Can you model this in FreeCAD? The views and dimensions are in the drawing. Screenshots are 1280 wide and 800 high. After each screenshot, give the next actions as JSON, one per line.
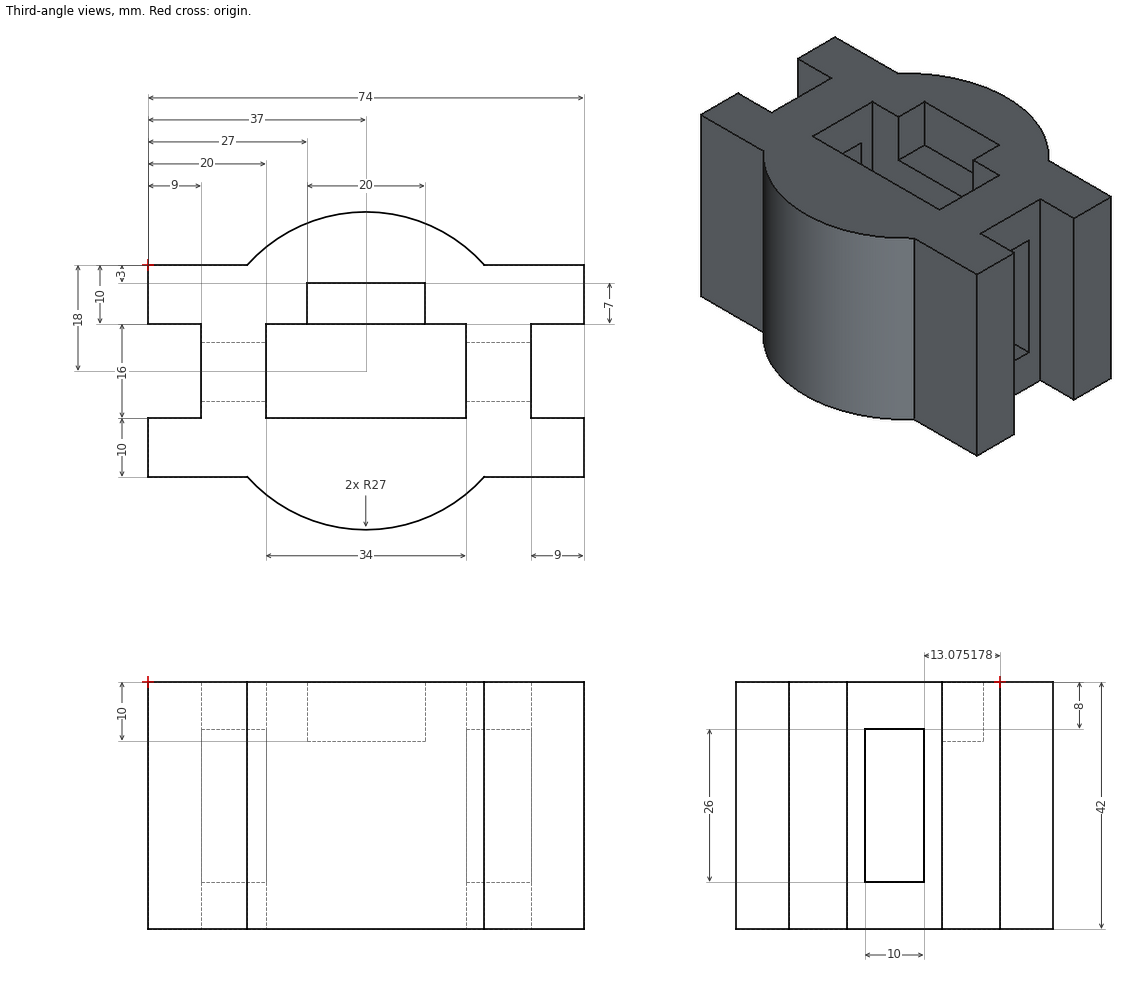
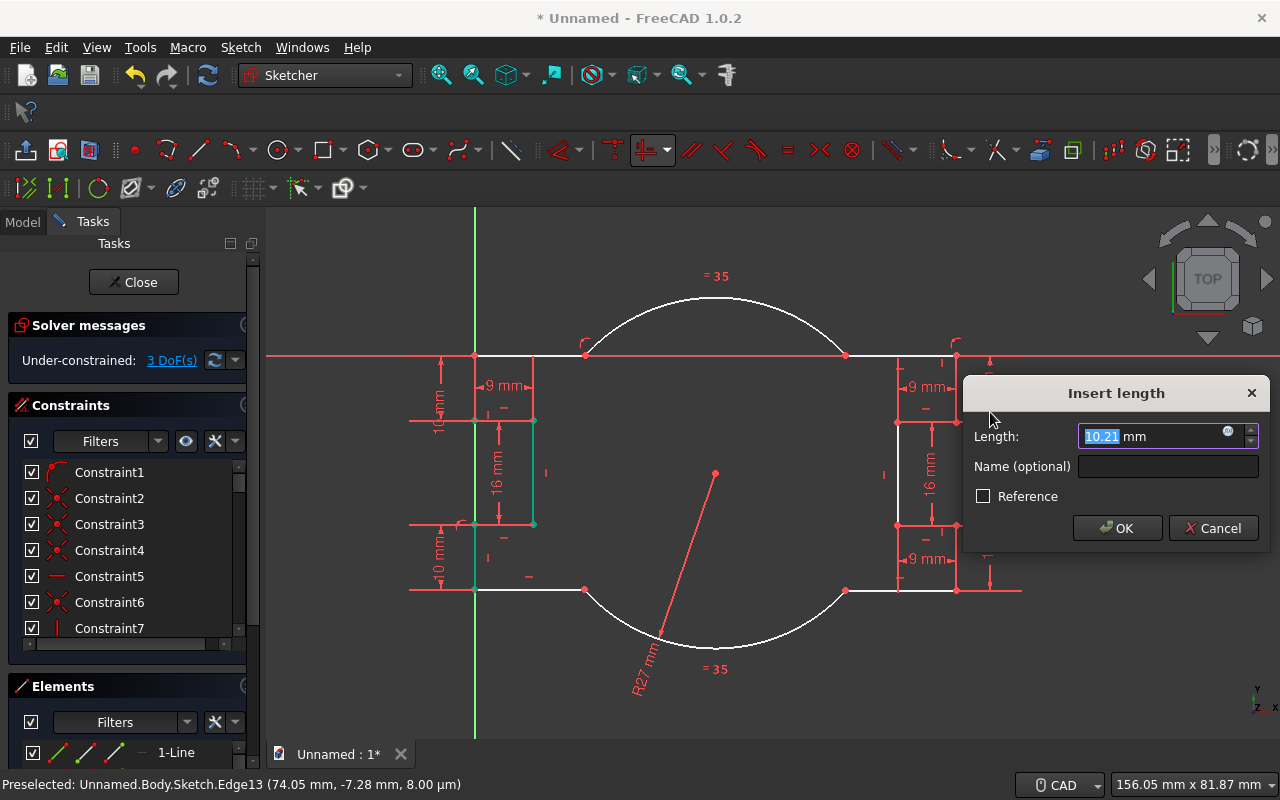
{"action": "type", "text": "10"}
{"action": "key", "text": "Return"}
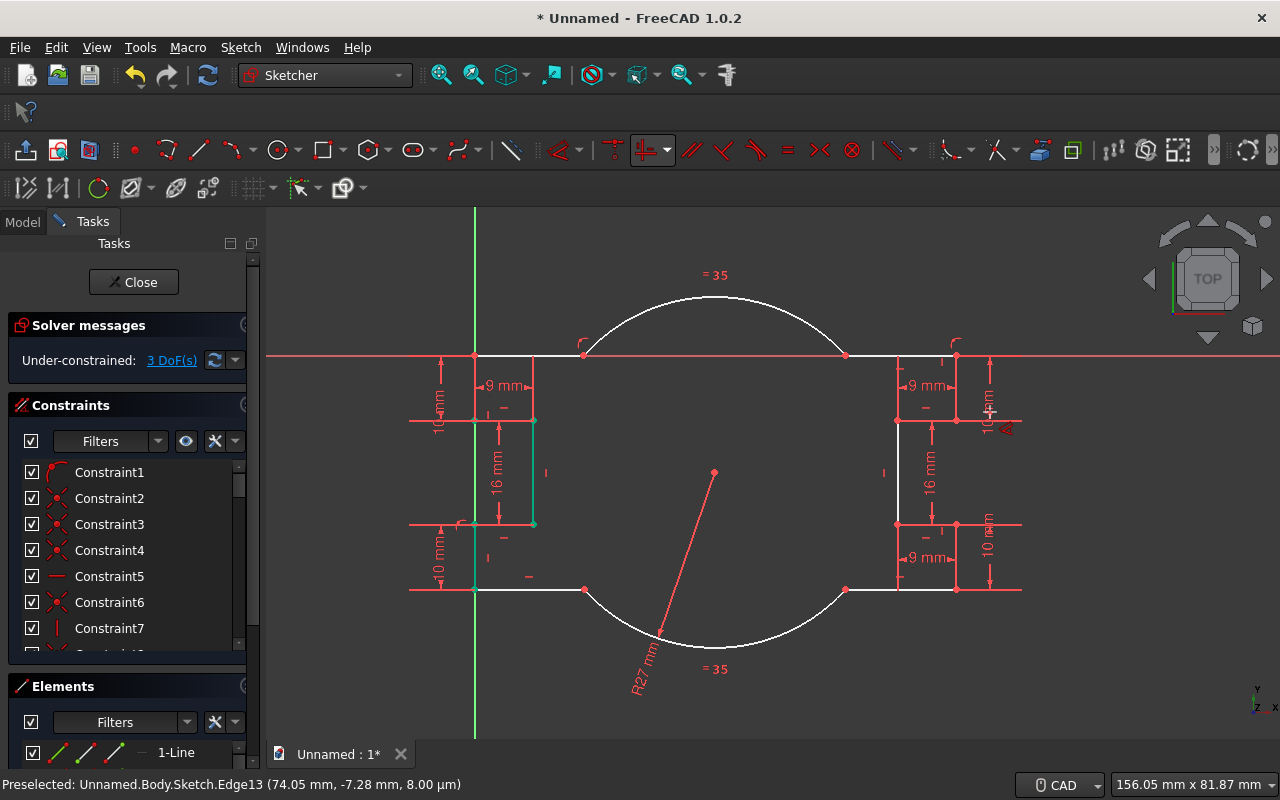
{"action": "left_click", "coordinate": [956, 590]}
{"action": "left_click", "coordinate": [715, 624]}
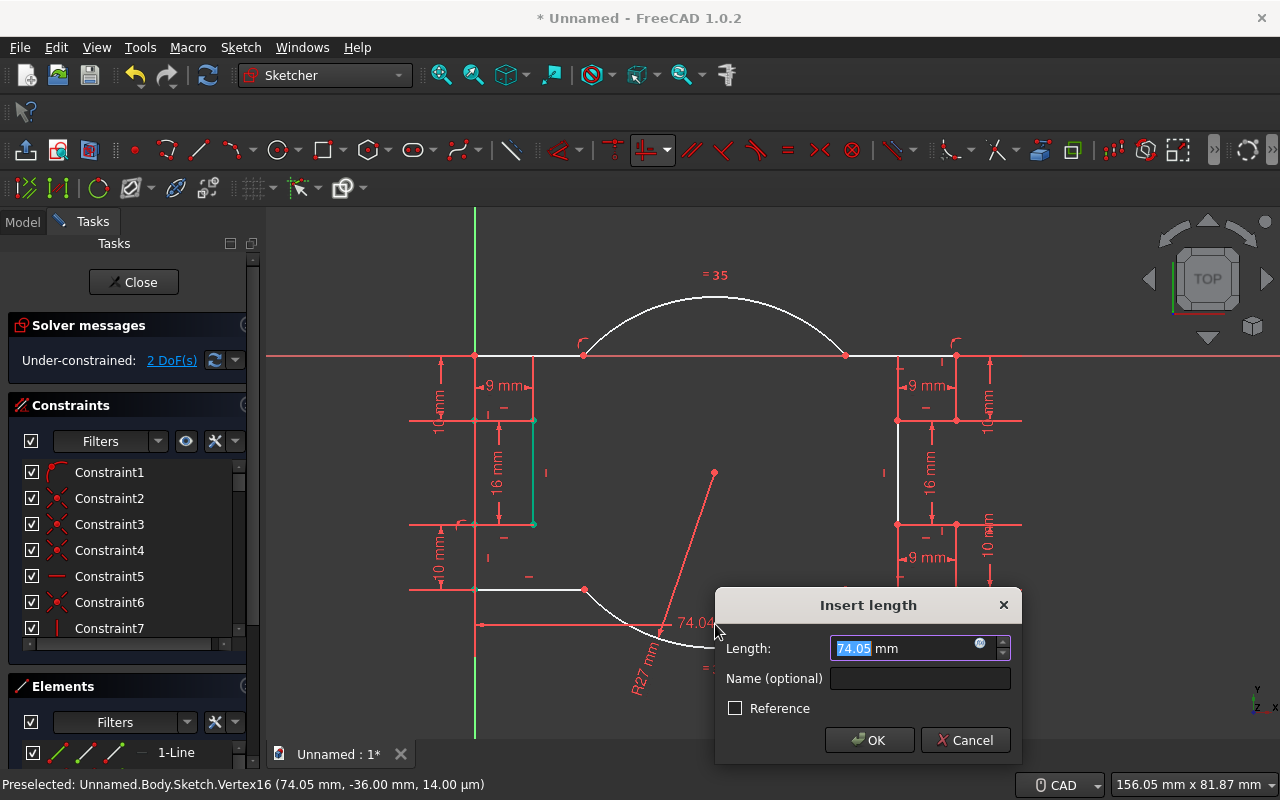
{"action": "type", "text": "74"}
{"action": "key", "text": "Return"}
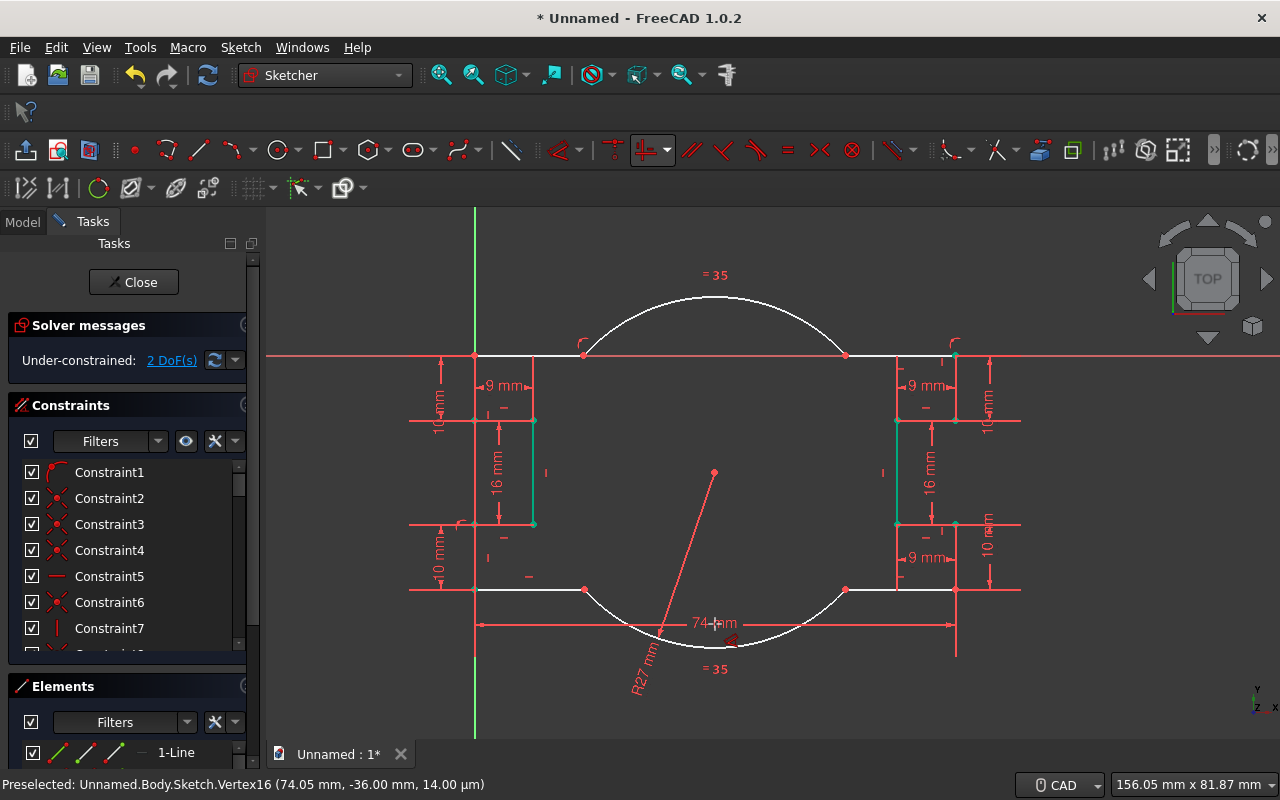
{"action": "left_click", "coordinate": [715, 472]}
{"action": "left_click", "coordinate": [595, 322]}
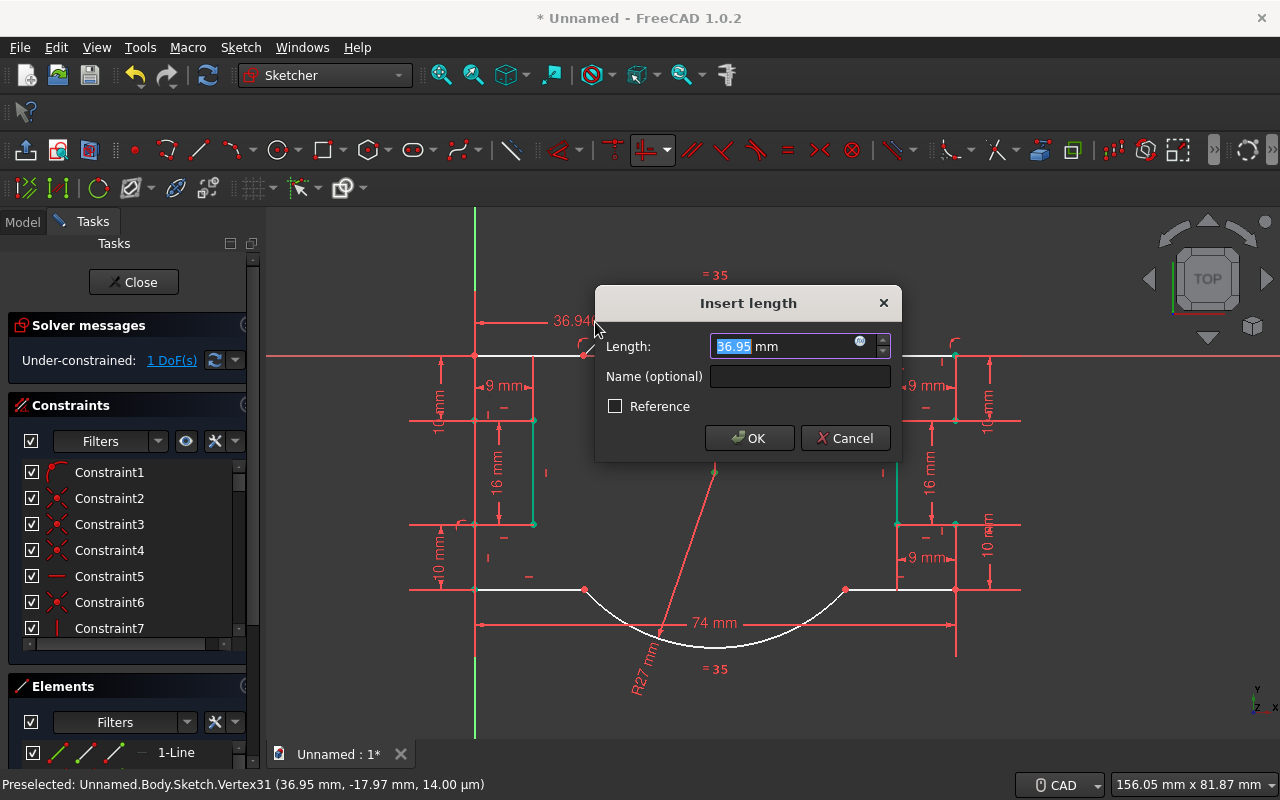
{"action": "type", "text": "37"}
{"action": "key", "text": "Return"}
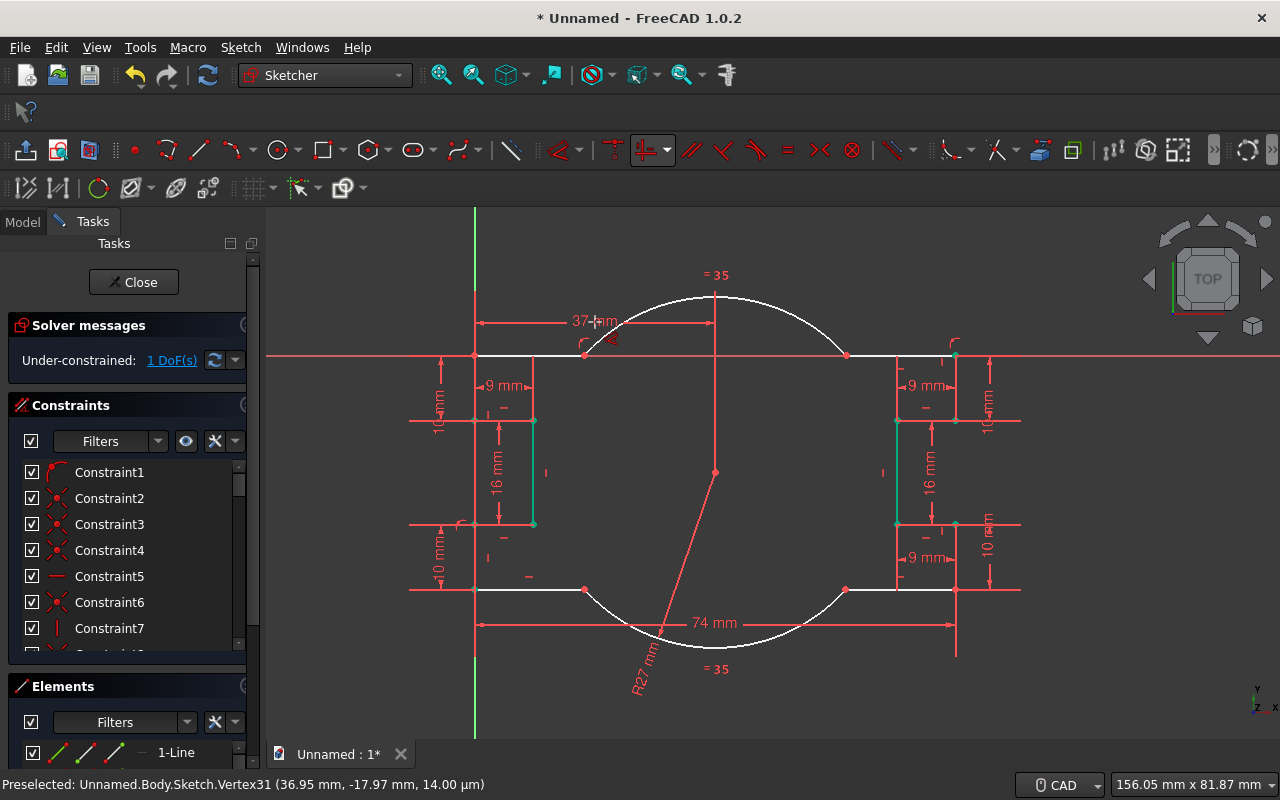
{"action": "left_click", "coordinate": [715, 472]}
{"action": "left_click", "coordinate": [441, 441]}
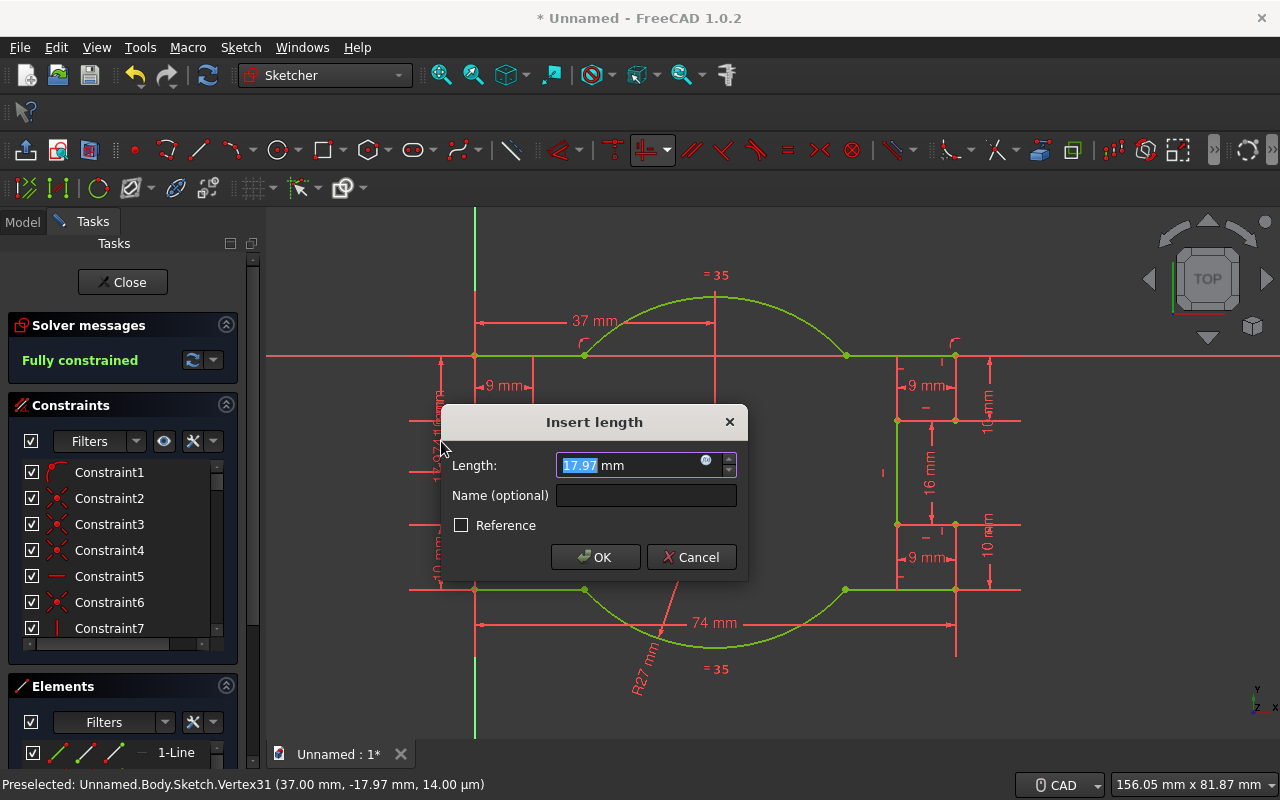
{"action": "type", "text": "18"}
{"action": "key", "text": "Return"}
{"action": "key", "text": "Escape"}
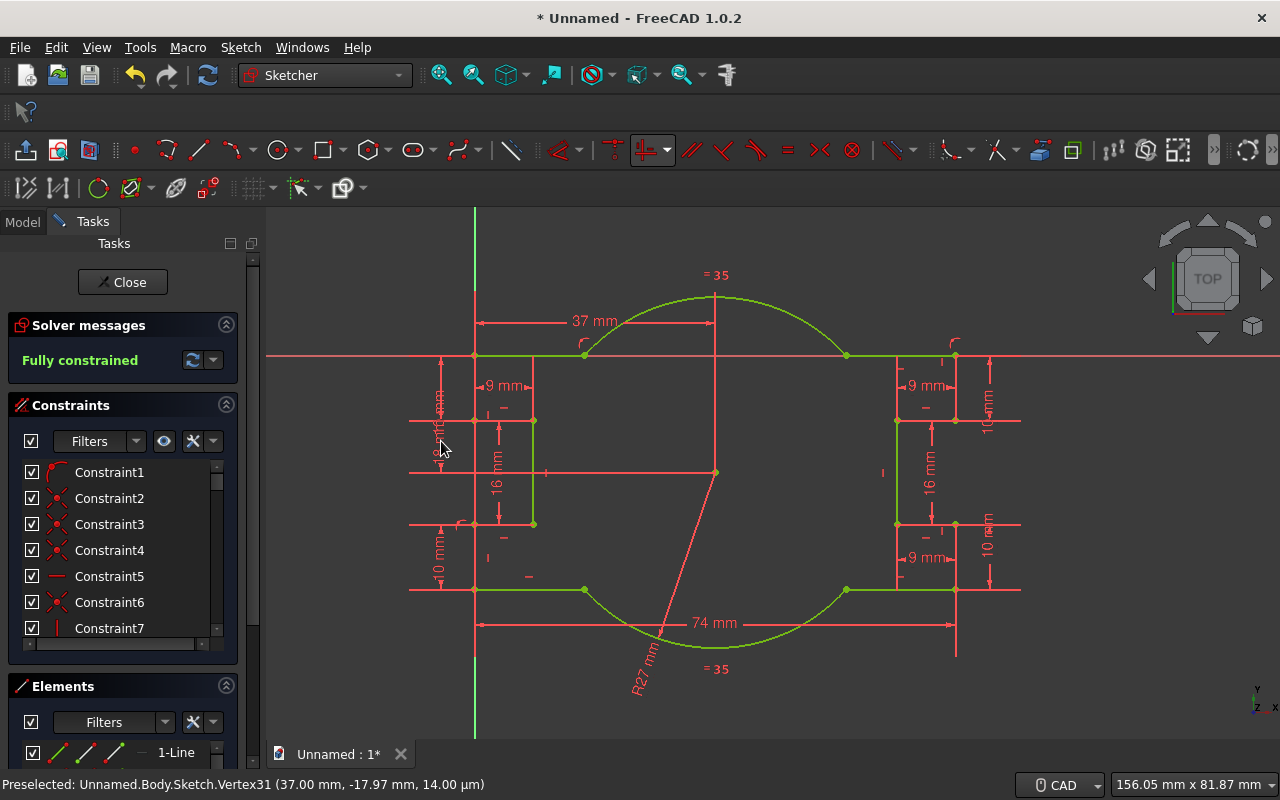
{"action": "left_click", "coordinate": [123, 282]}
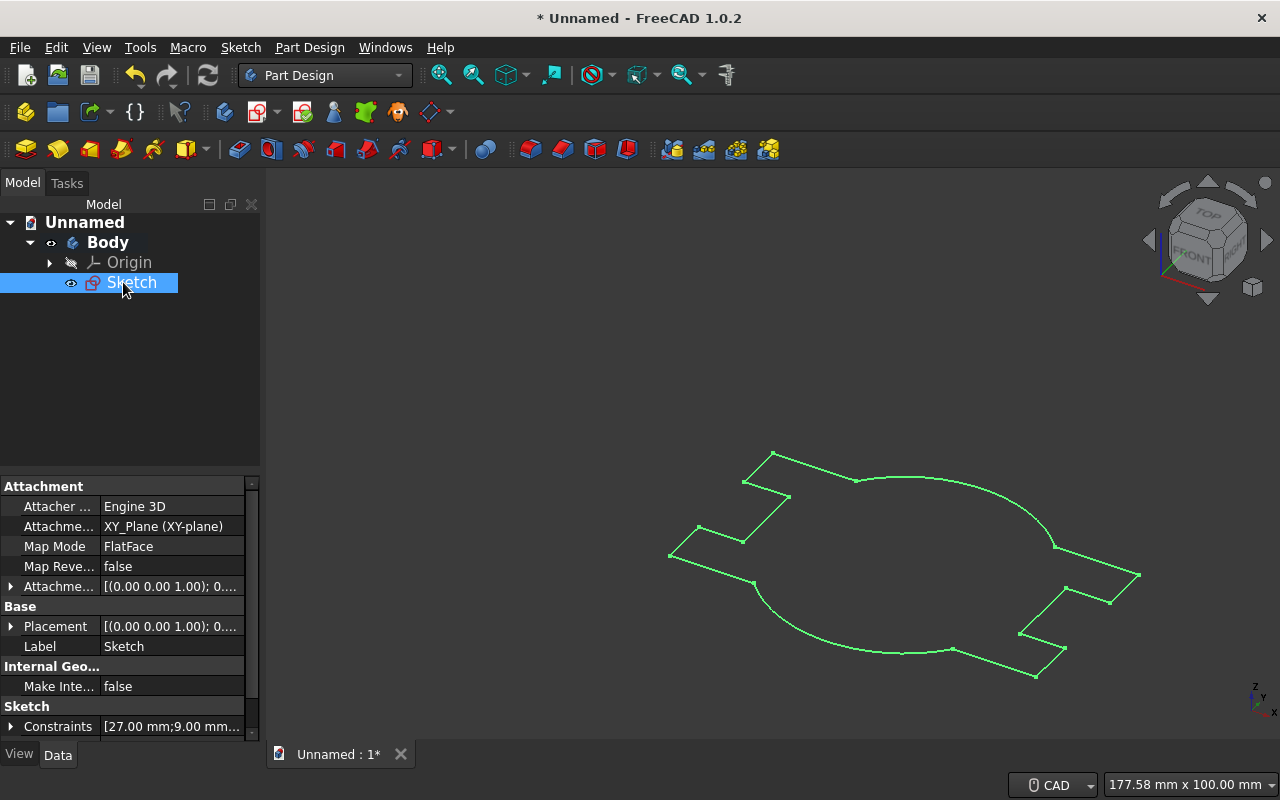
{"action": "left_click", "coordinate": [26, 150]}